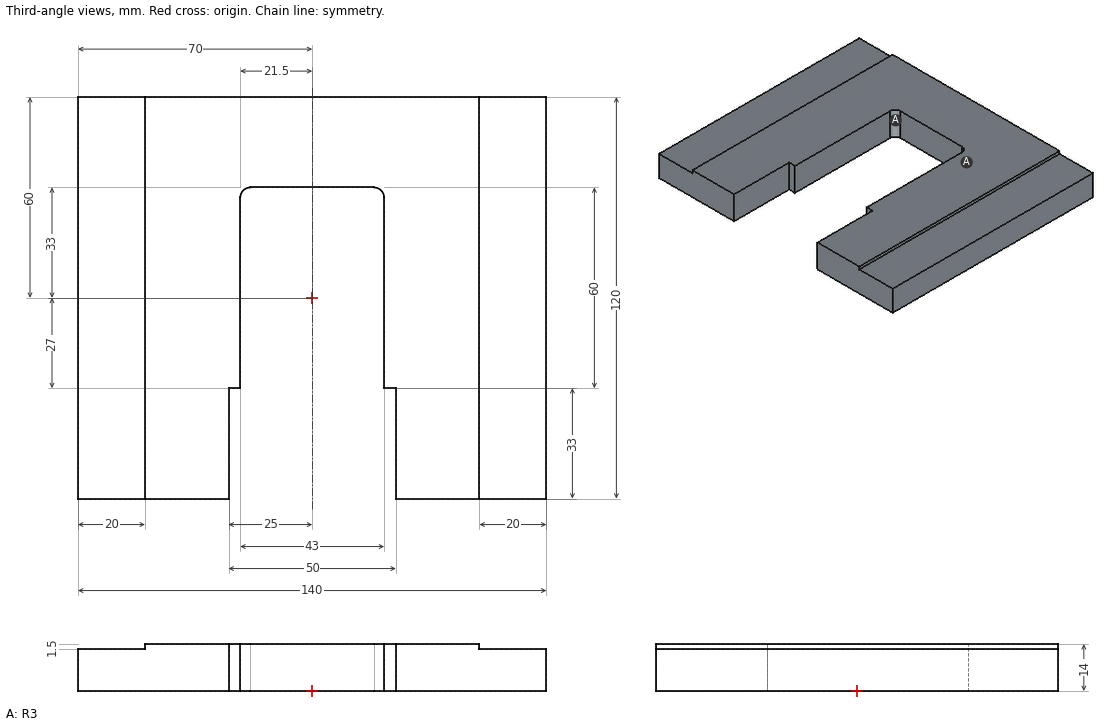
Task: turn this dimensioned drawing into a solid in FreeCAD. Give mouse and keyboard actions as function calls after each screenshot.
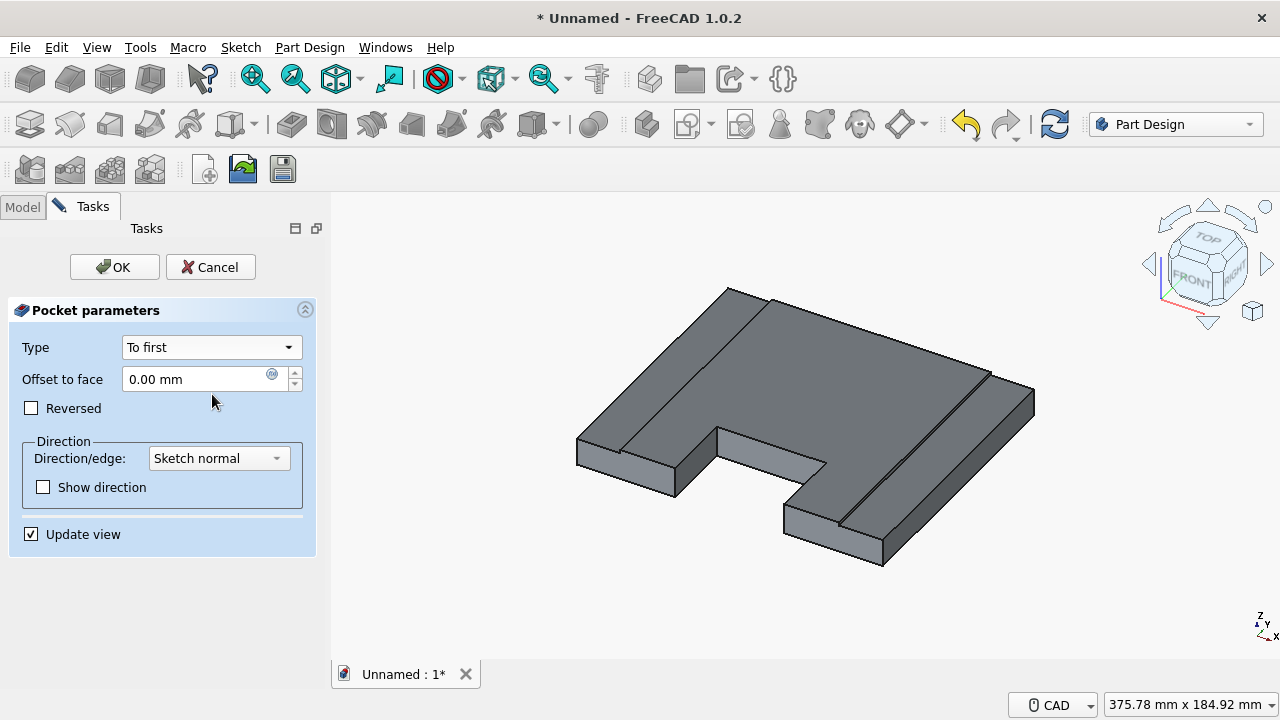
click(115, 267)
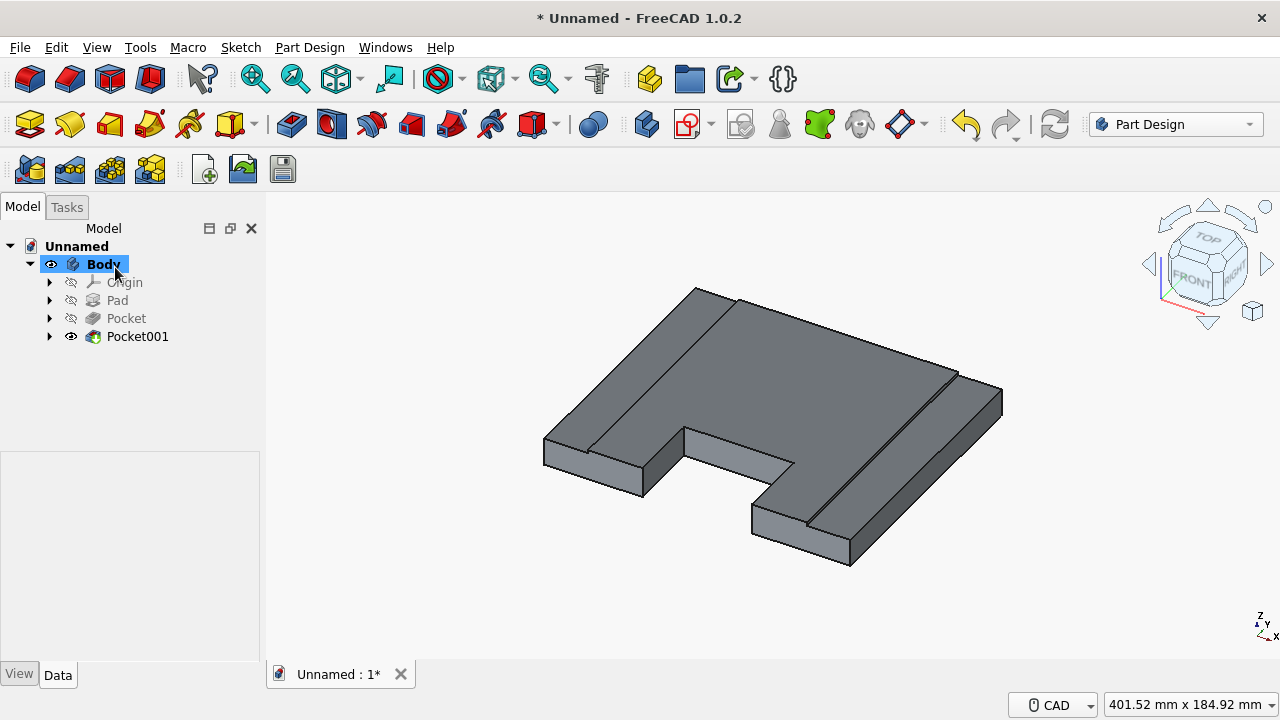
click(688, 124)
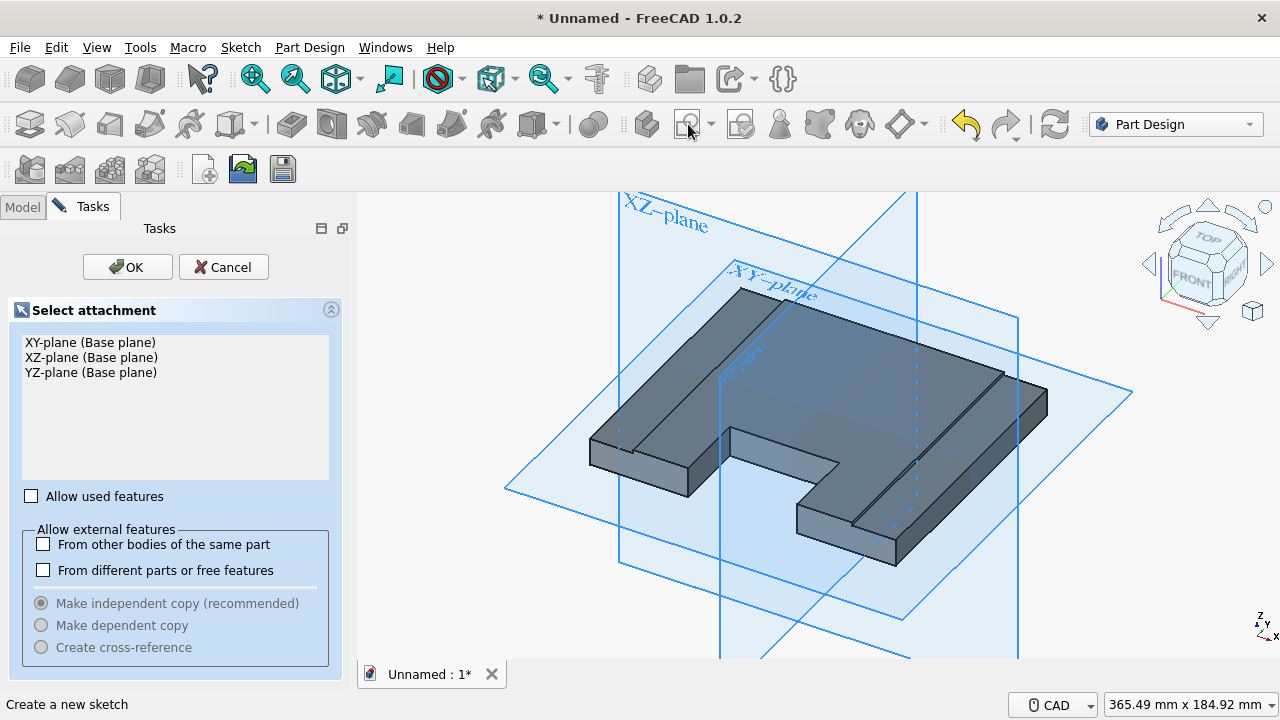
click(82, 342)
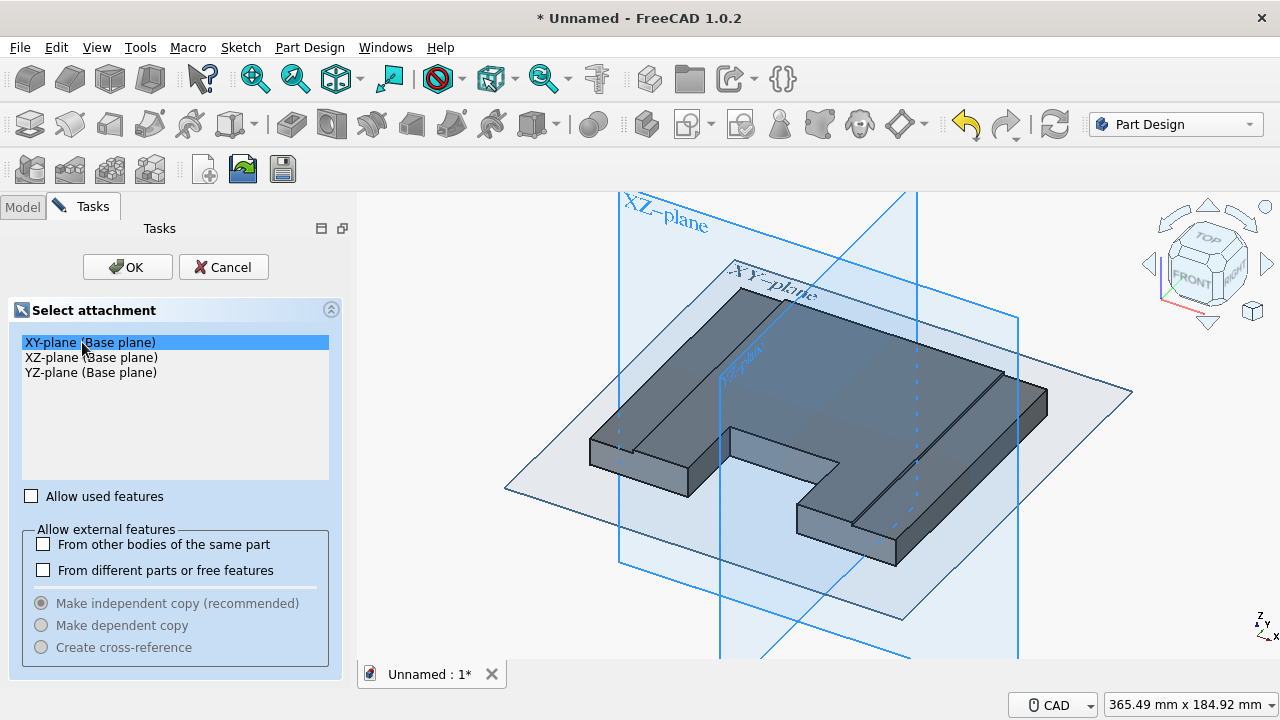
click(128, 267)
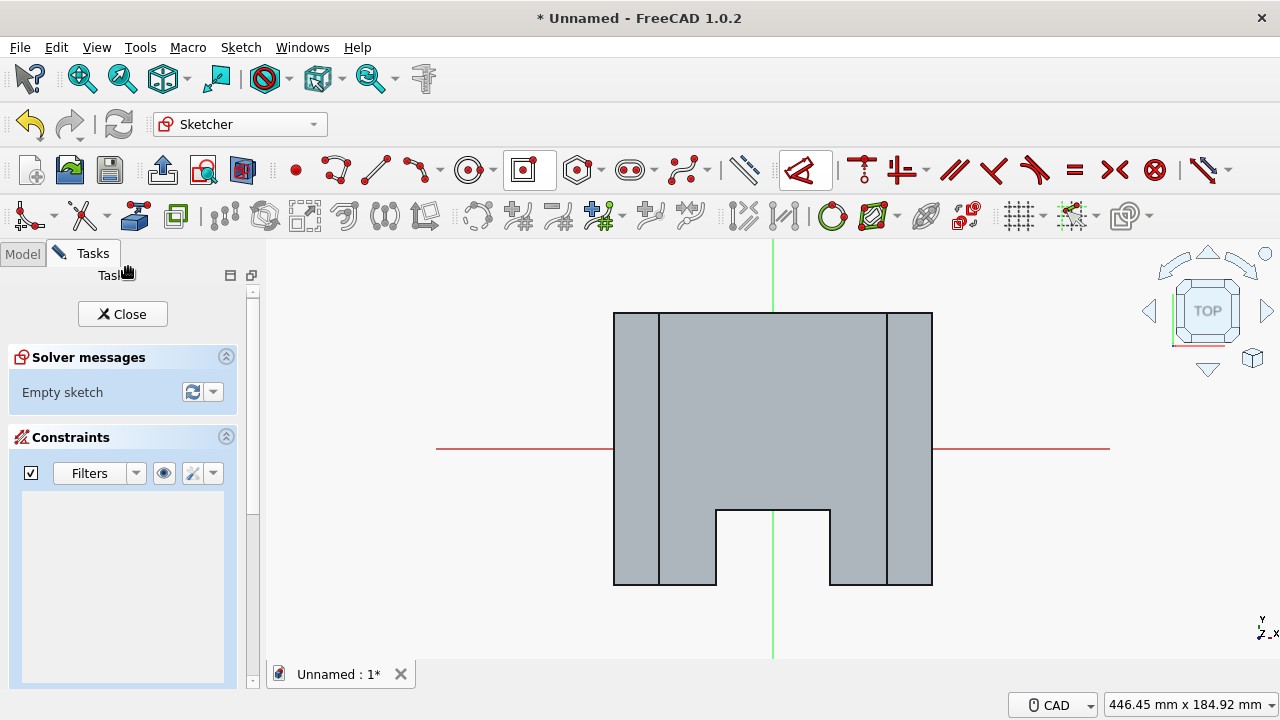
click(244, 170)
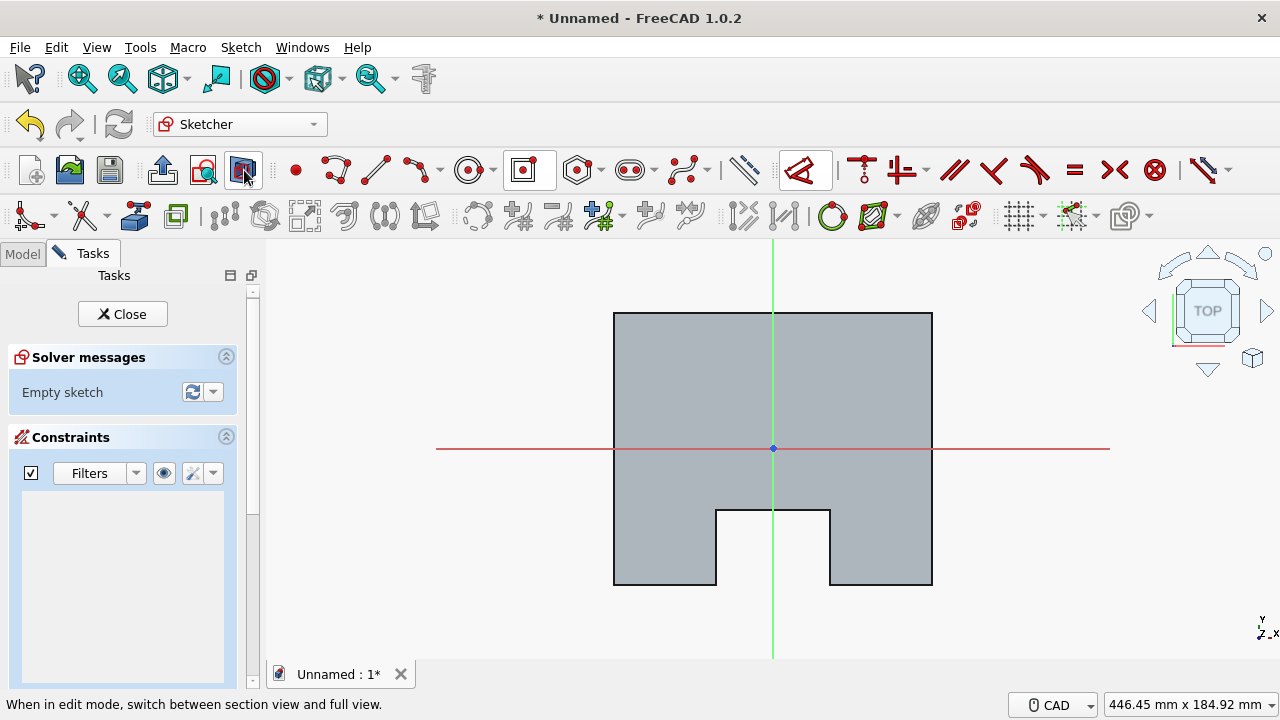
scroll(856, 434, up, 3)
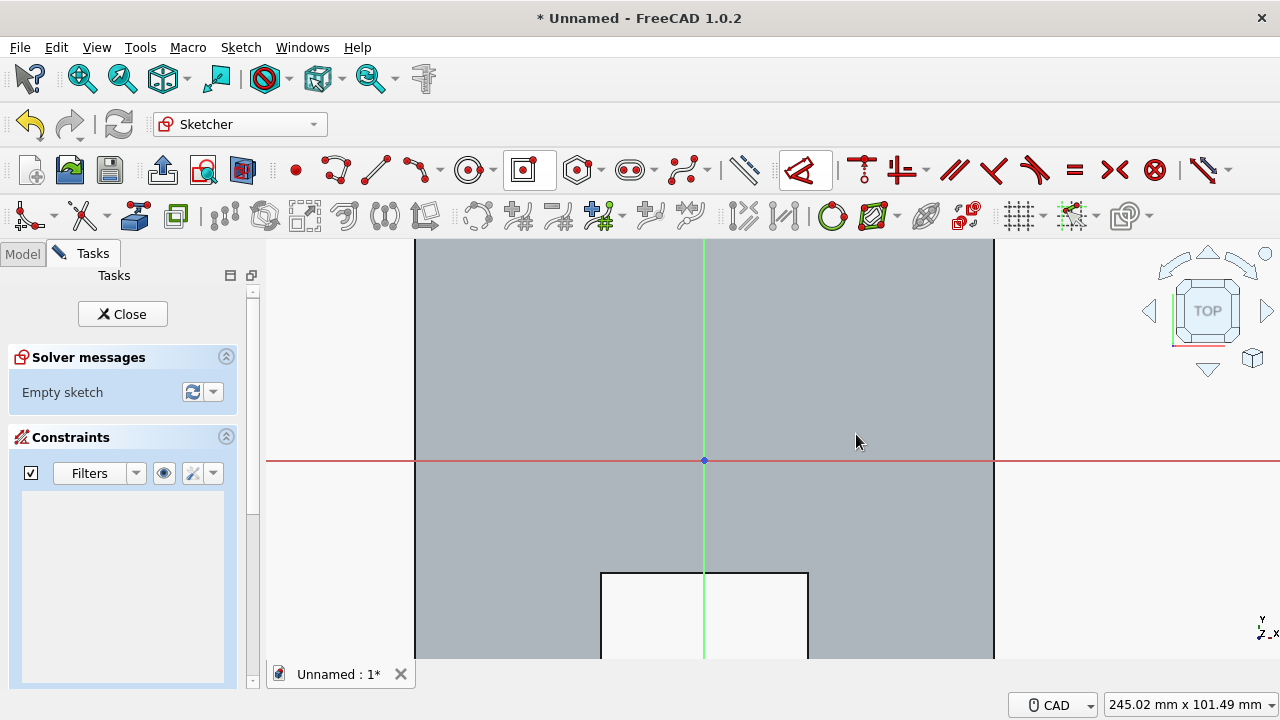
key(g)
key(r)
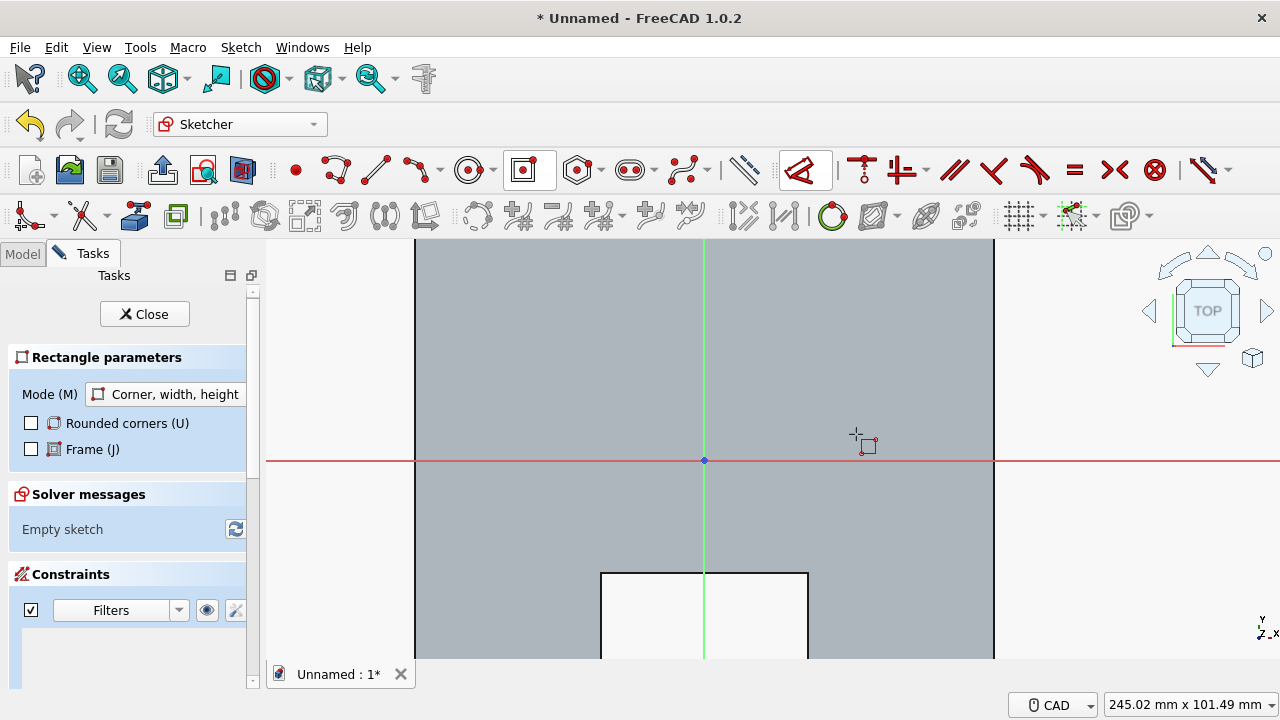
click(615, 324)
move(793, 573)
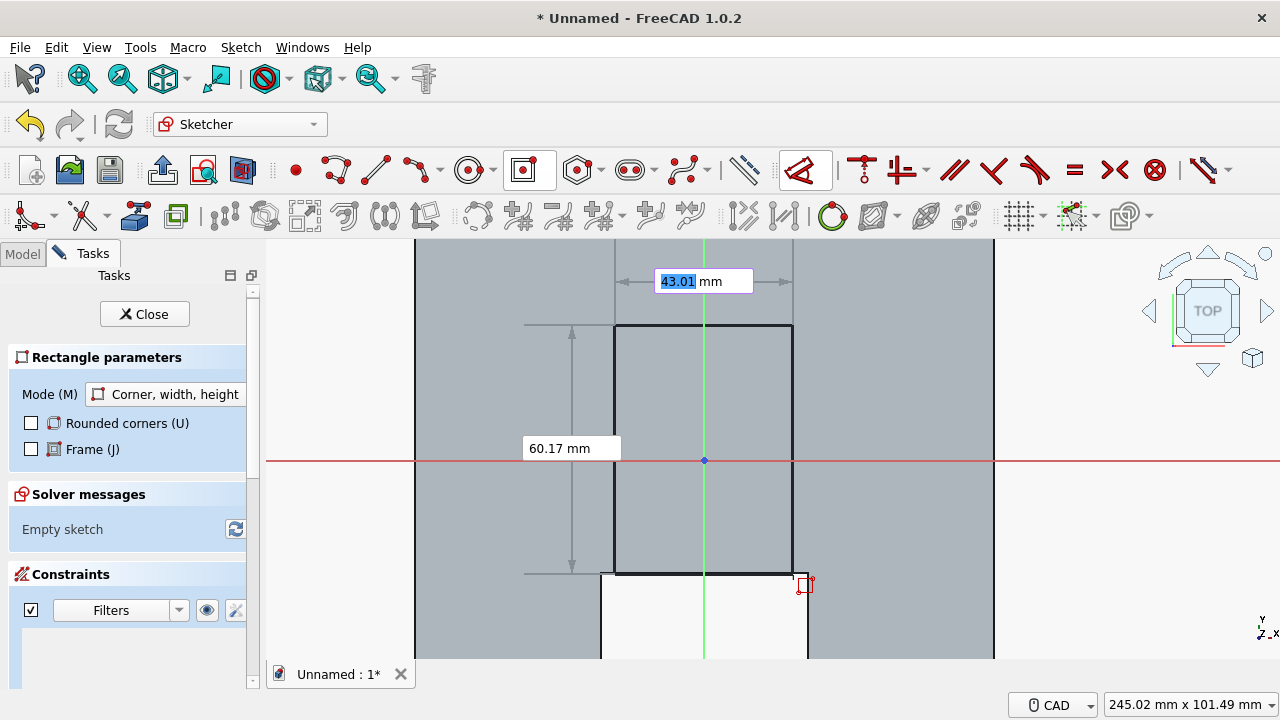
text(43)
key(Tab)
text(60)
key(Return)
key(Escape)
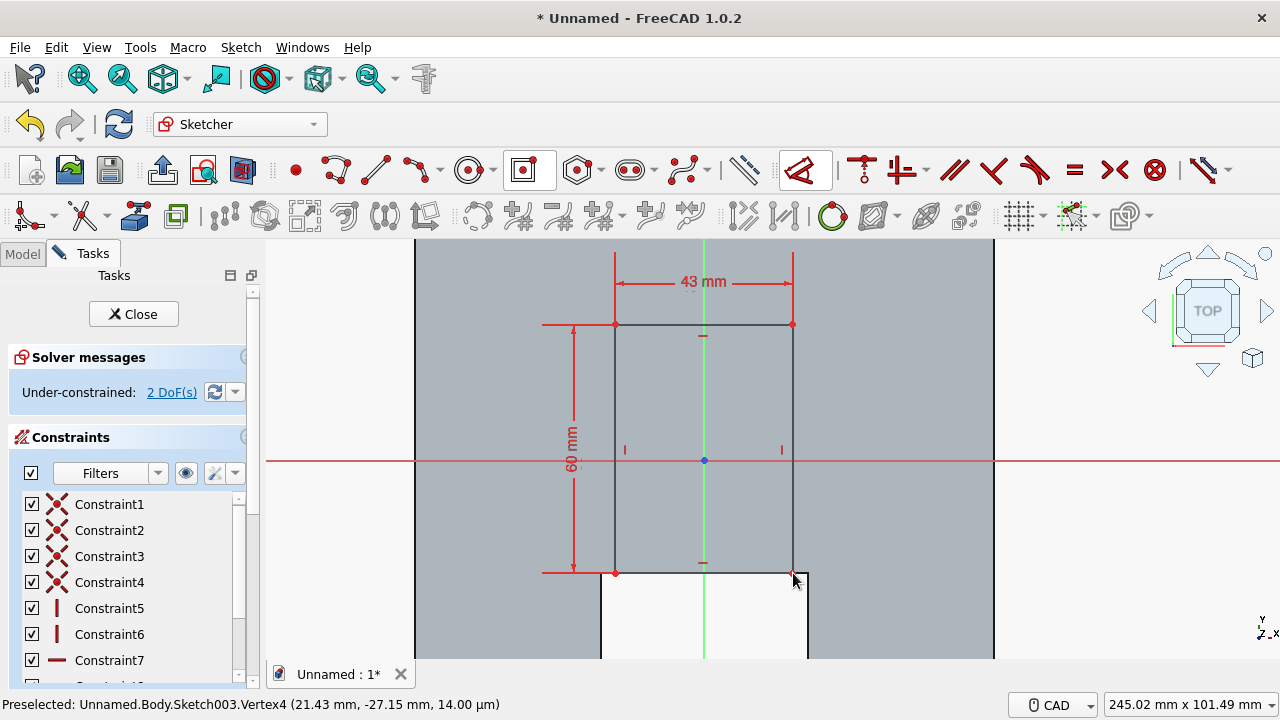
click(615, 325)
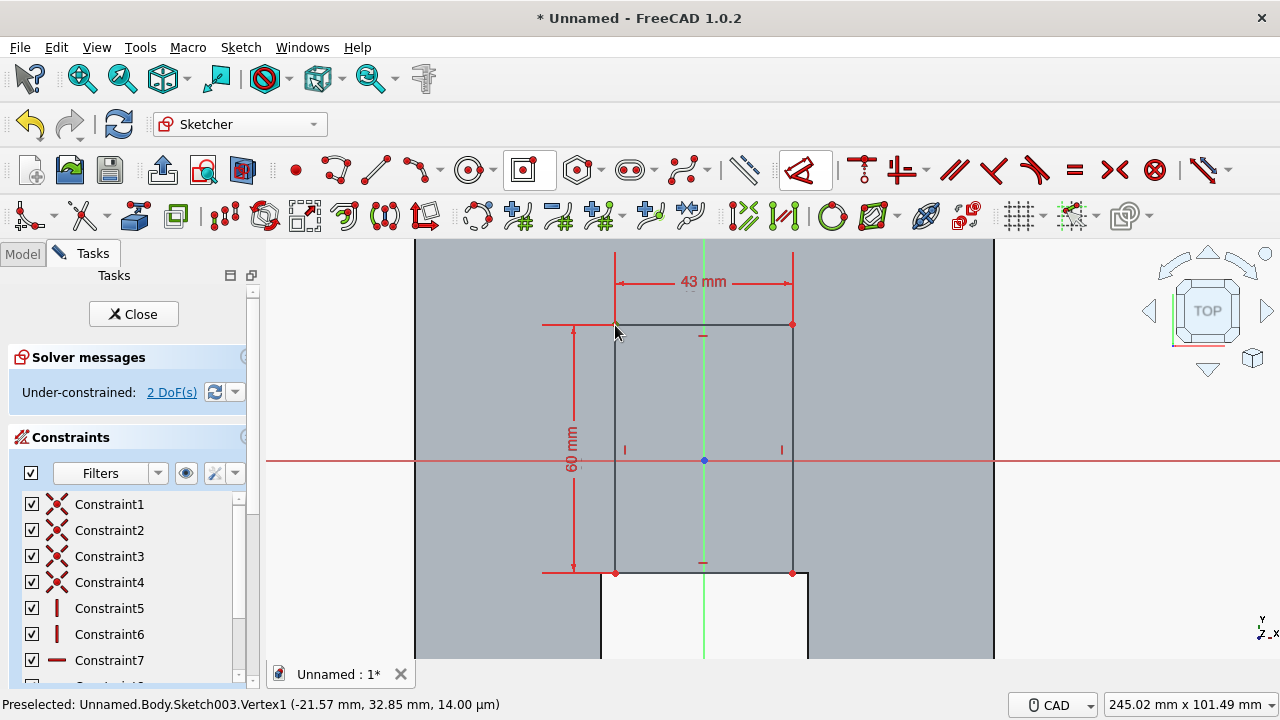
key(i)